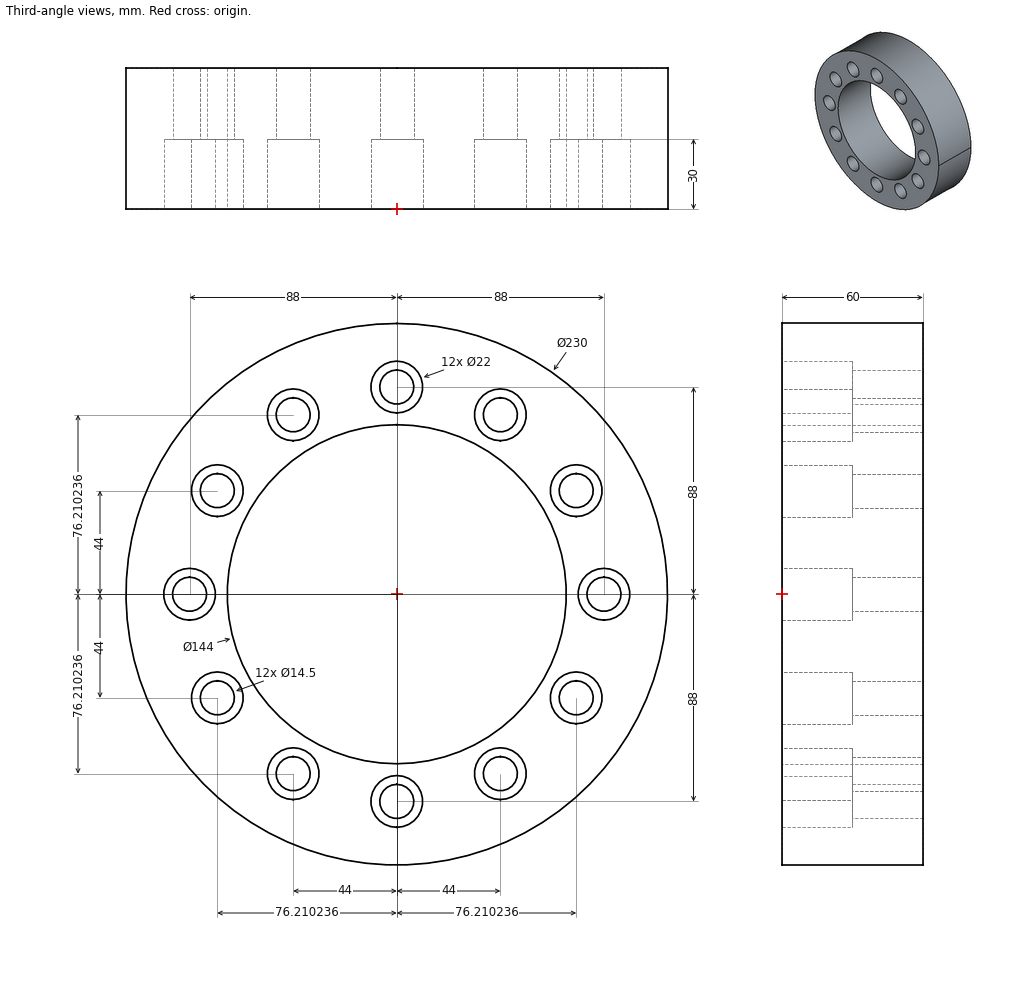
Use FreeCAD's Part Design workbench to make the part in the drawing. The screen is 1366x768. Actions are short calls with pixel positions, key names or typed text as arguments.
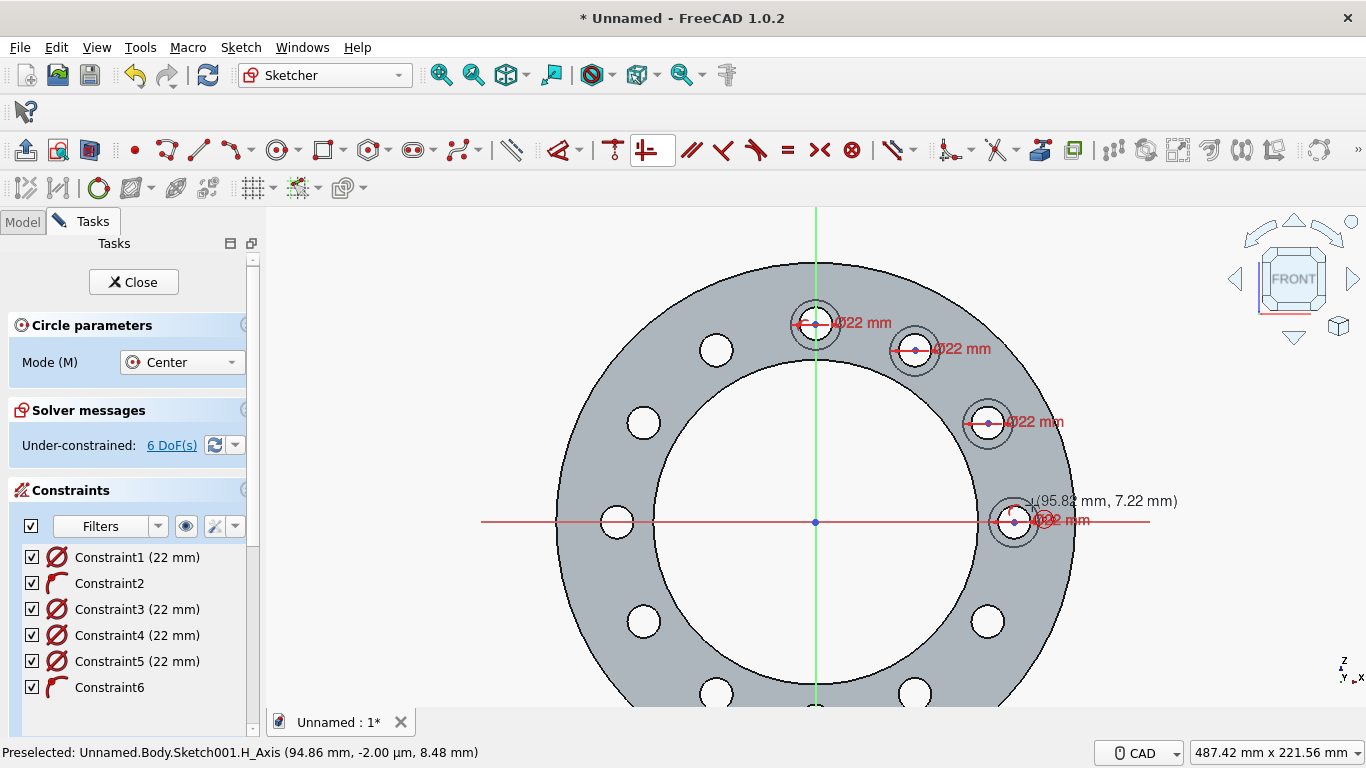
click(988, 622)
move(1005, 604)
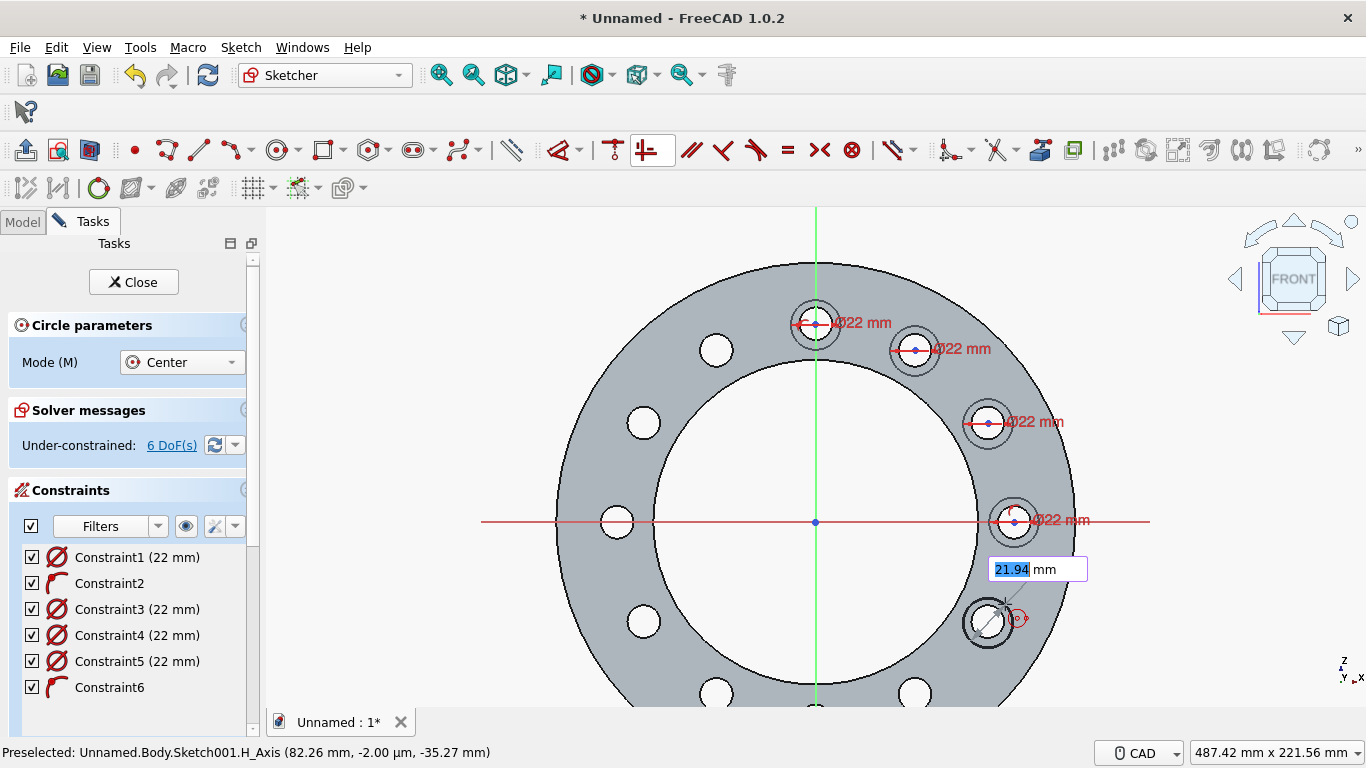
text(22)
key(Return)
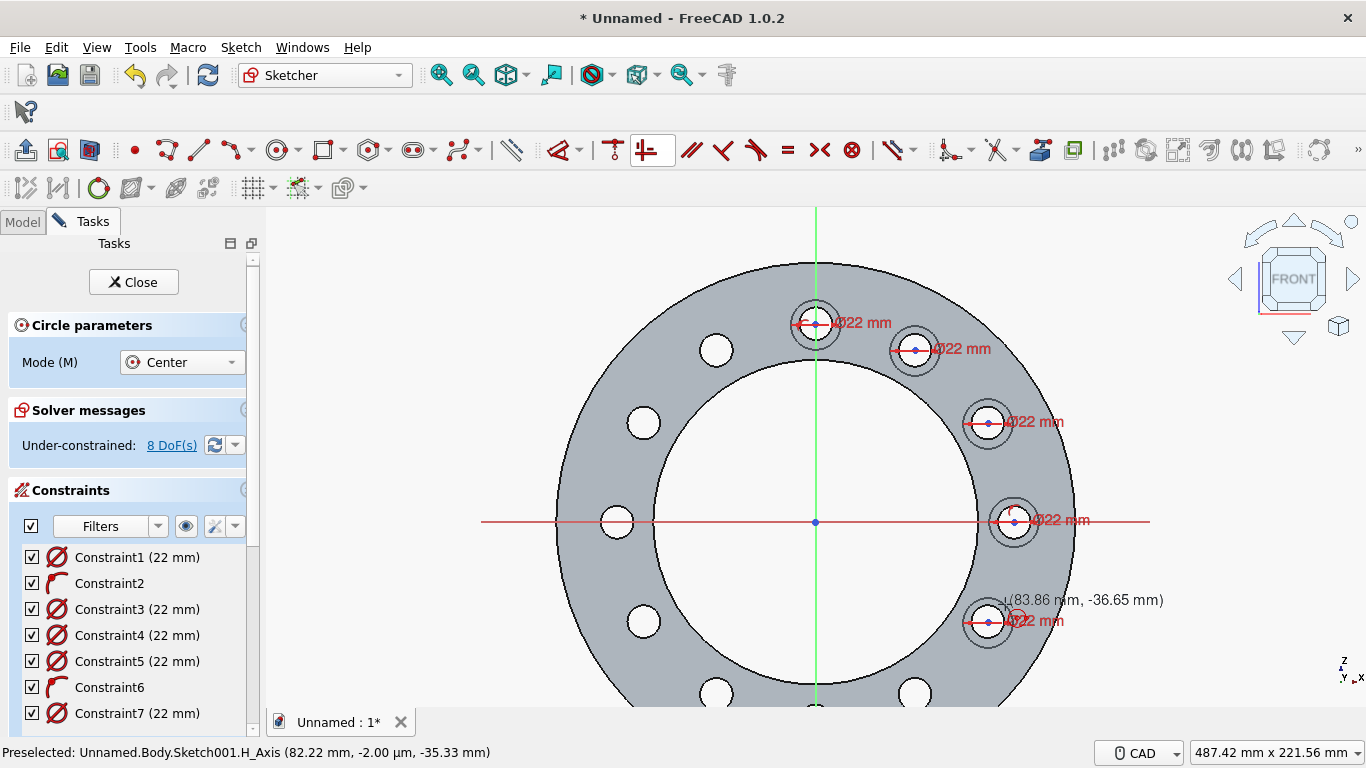
scroll(609, 324, down, 2)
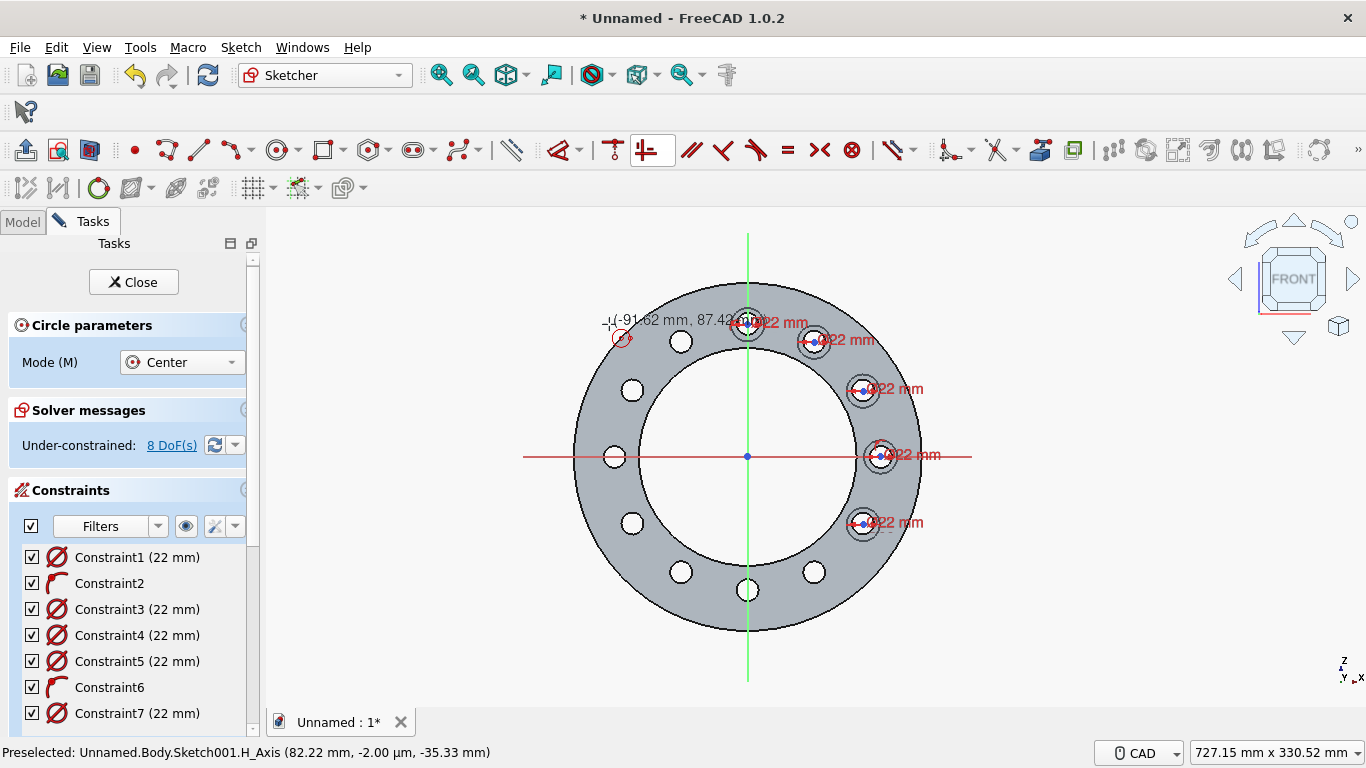
scroll(814, 572, up, 2)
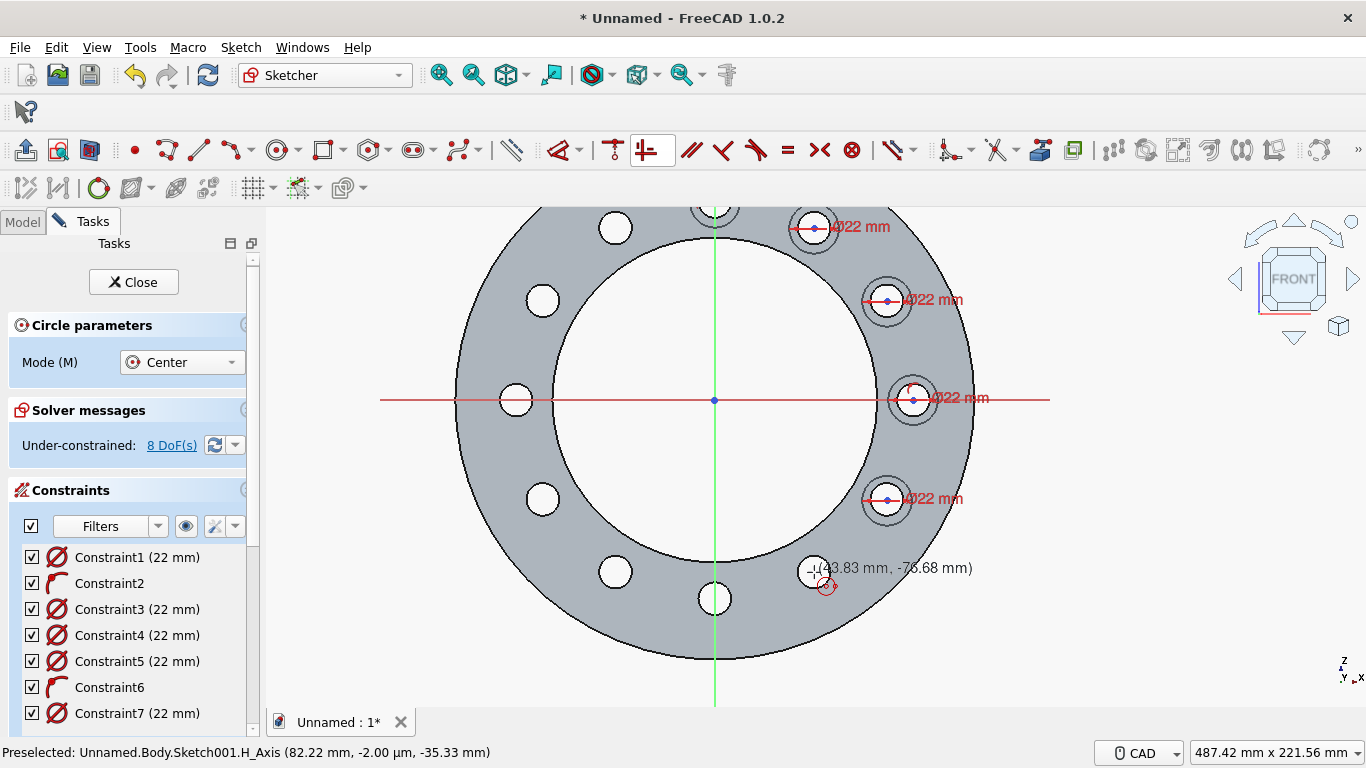
click(814, 572)
move(832, 555)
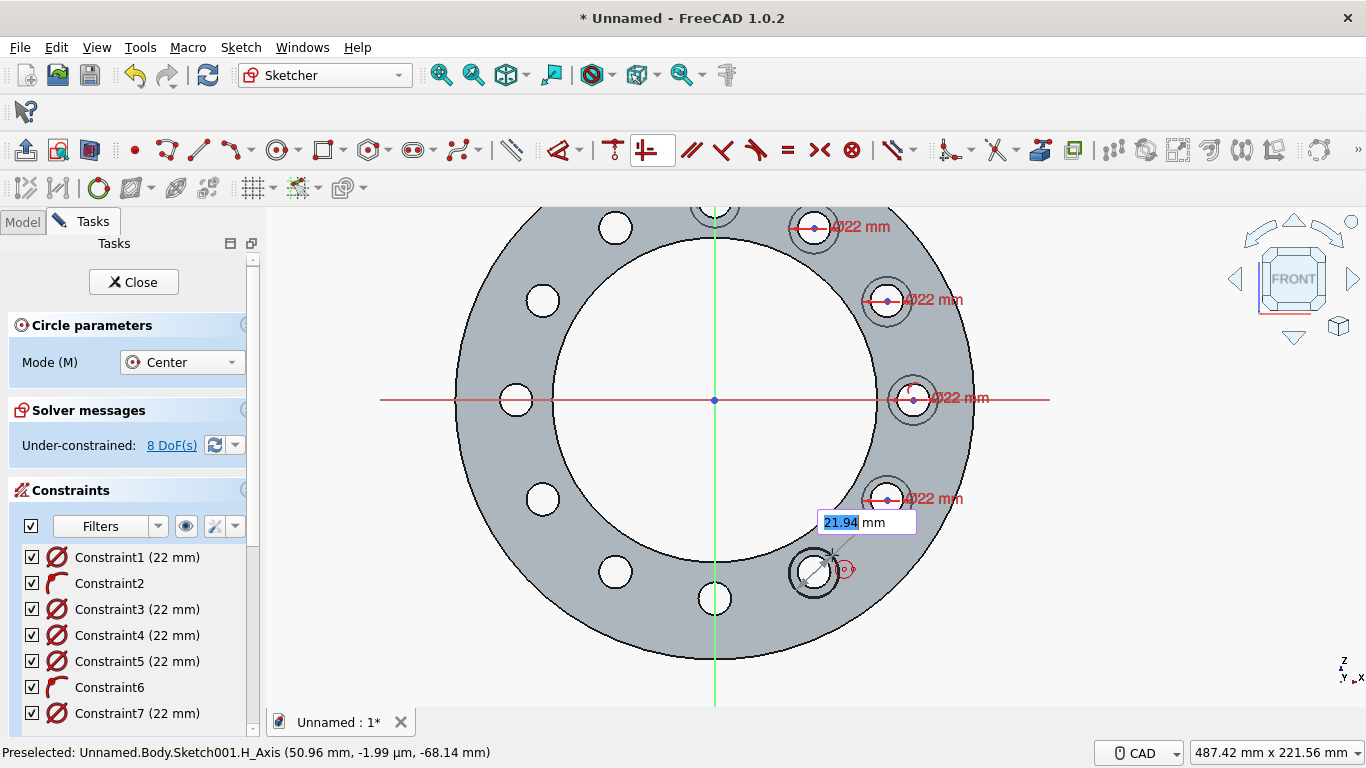
text(22)
key(Return)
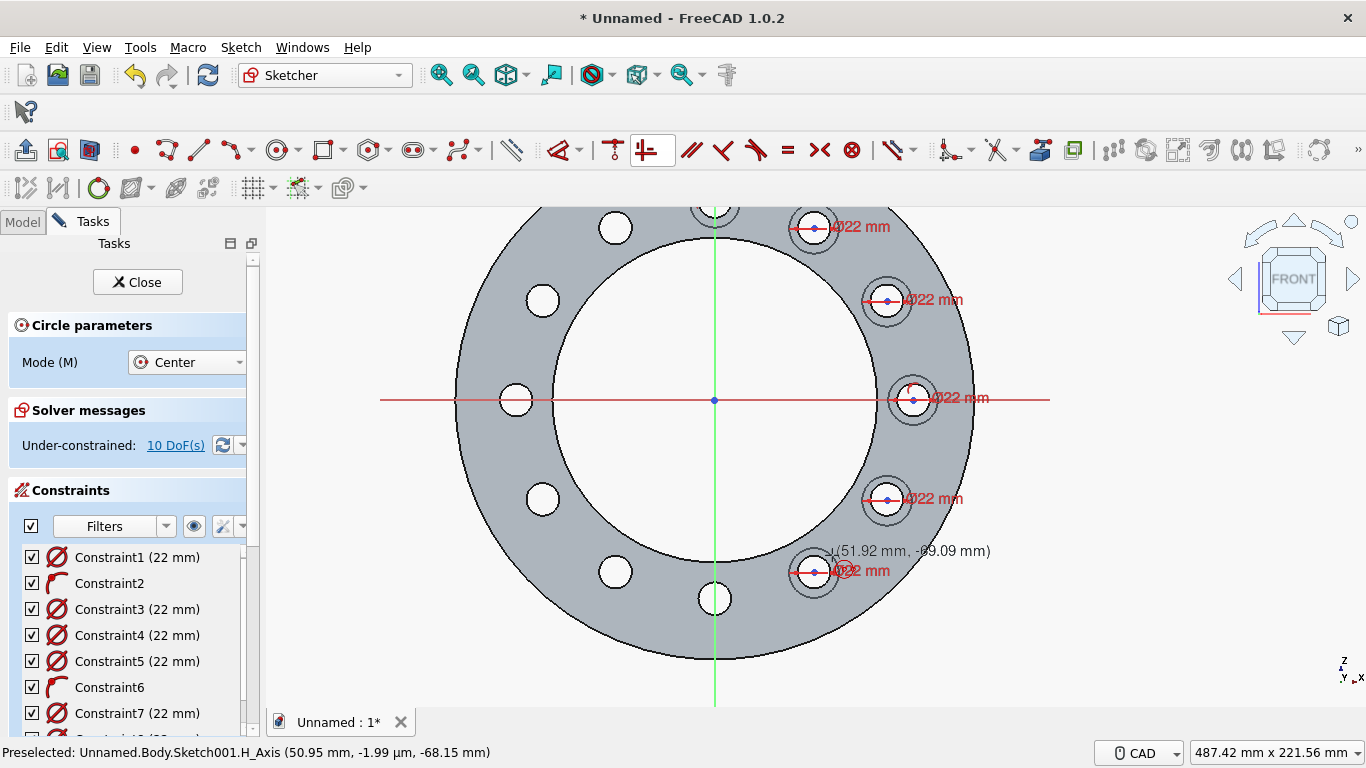
click(715, 599)
move(732, 581)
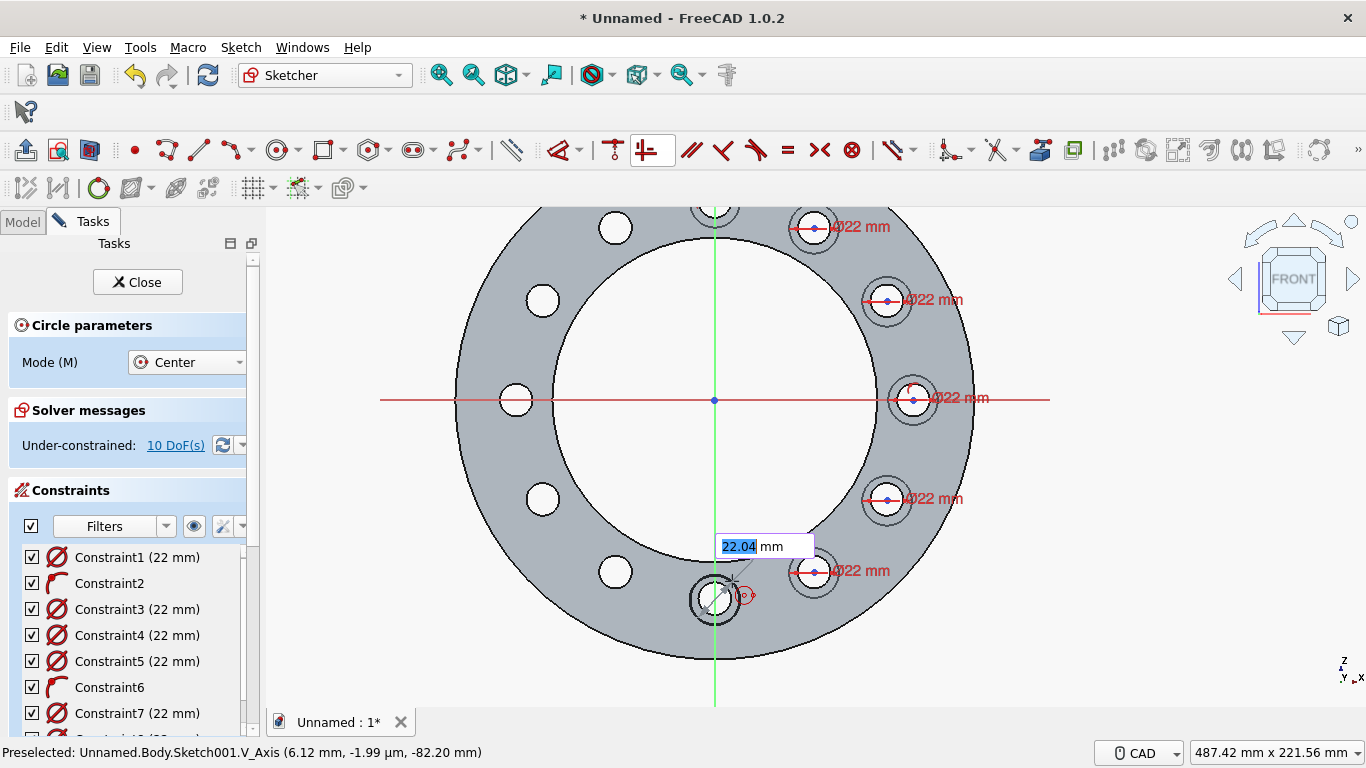
text(22)
key(Return)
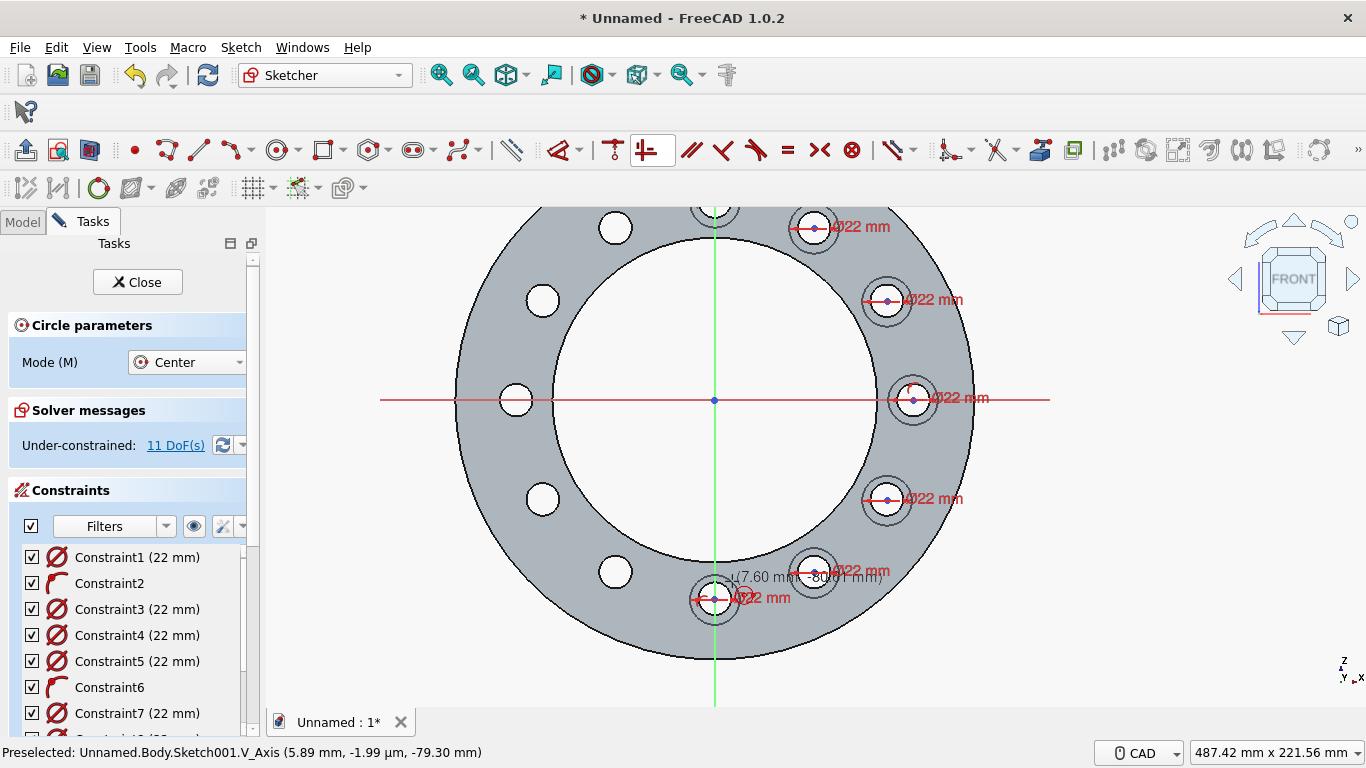
click(616, 572)
move(633, 555)